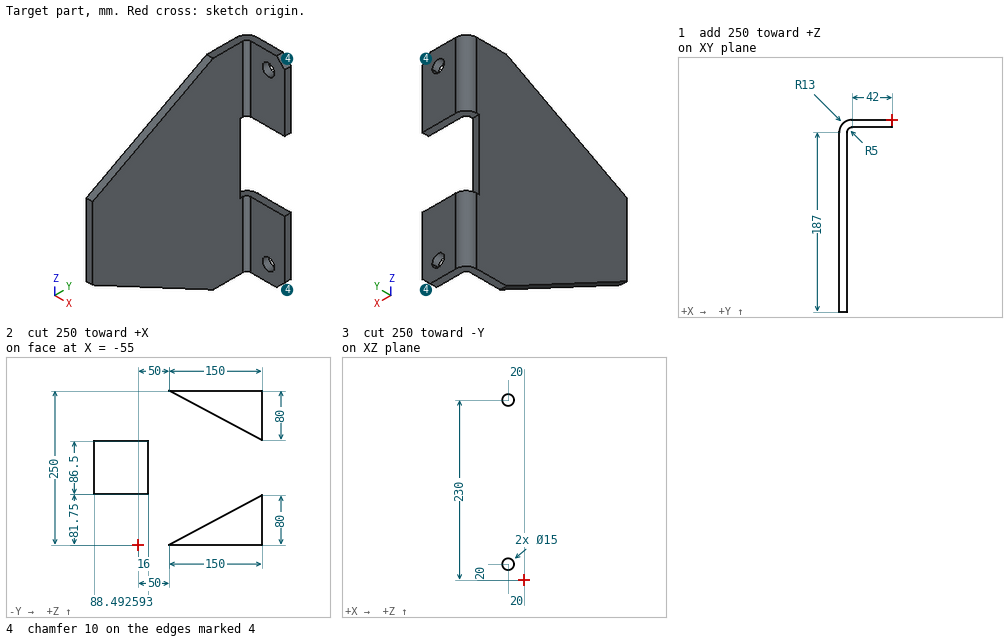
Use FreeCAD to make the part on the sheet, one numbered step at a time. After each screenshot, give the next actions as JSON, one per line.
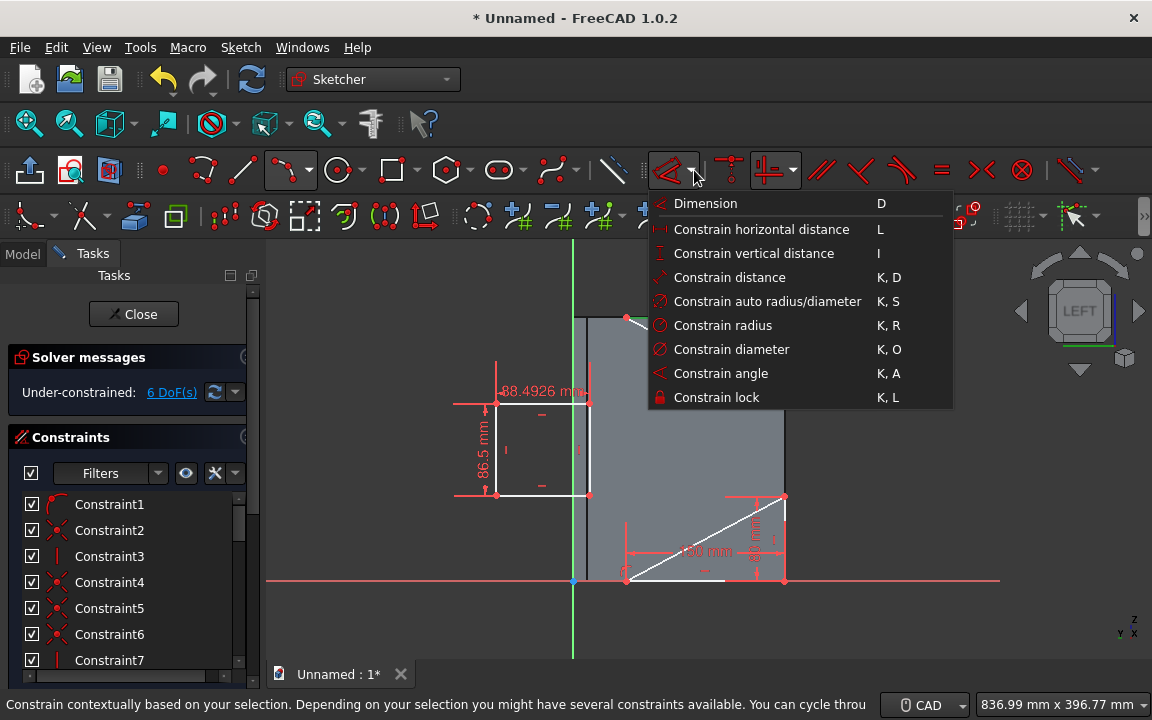
{"action": "left_click", "coordinate": [801, 229]}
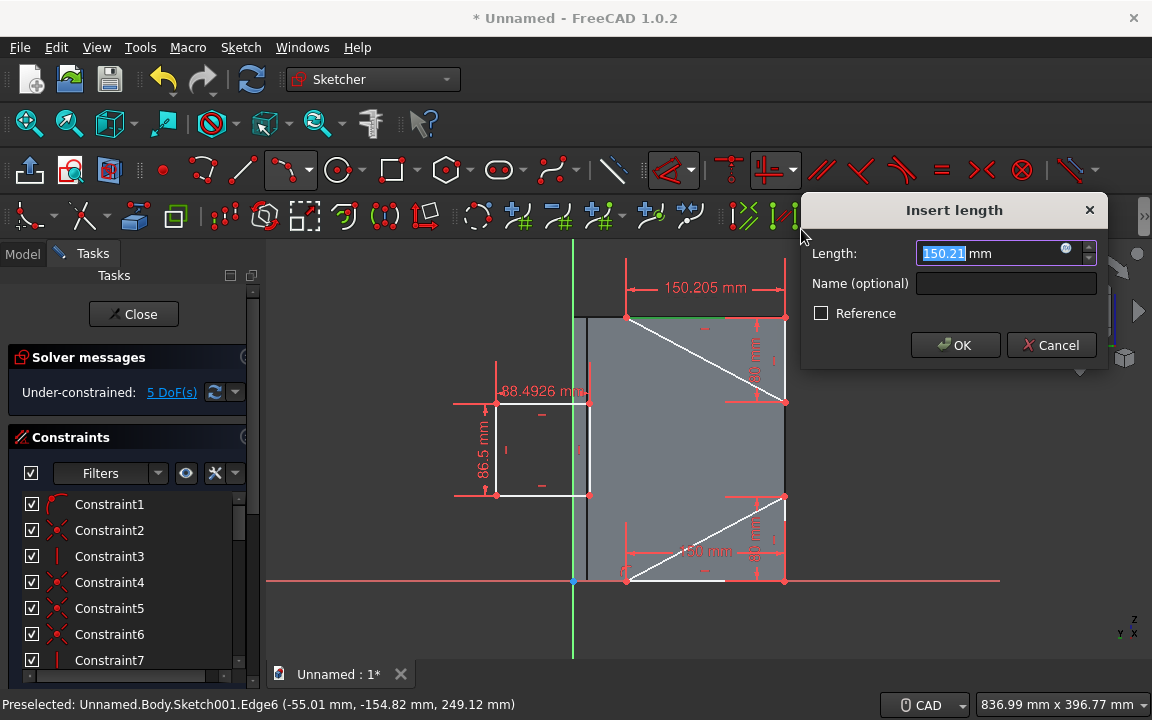
{"action": "type", "text": "150"}
{"action": "key", "text": "Return"}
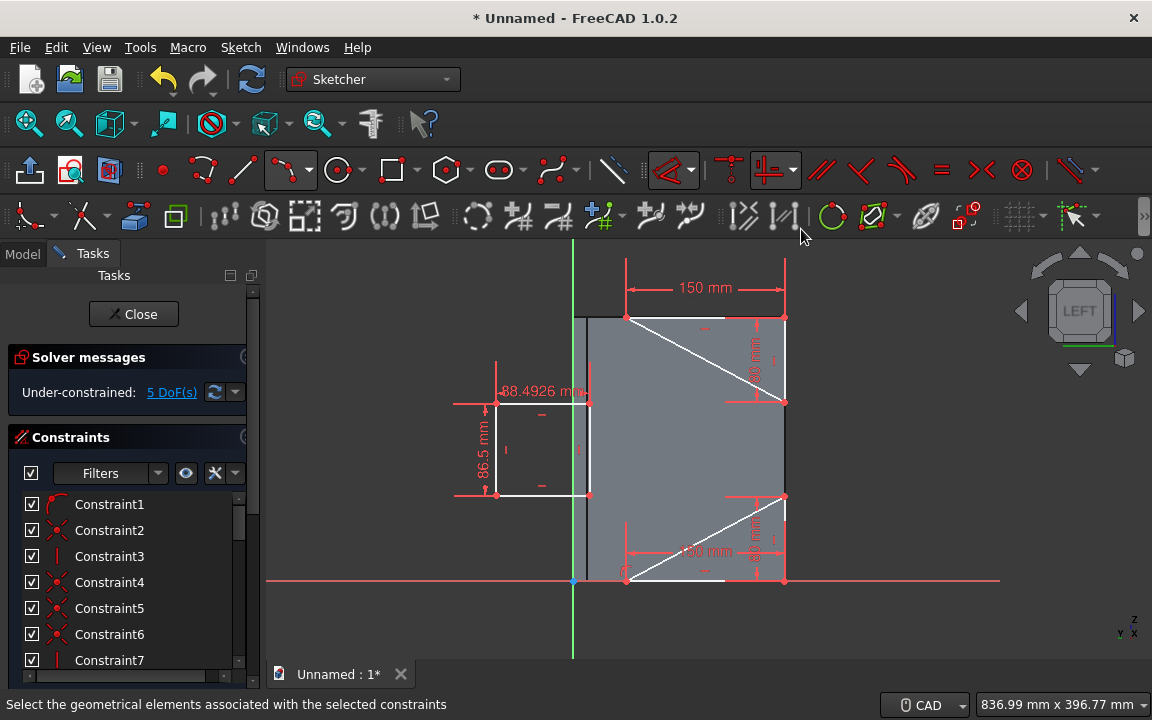
{"action": "left_click", "coordinate": [626, 581]}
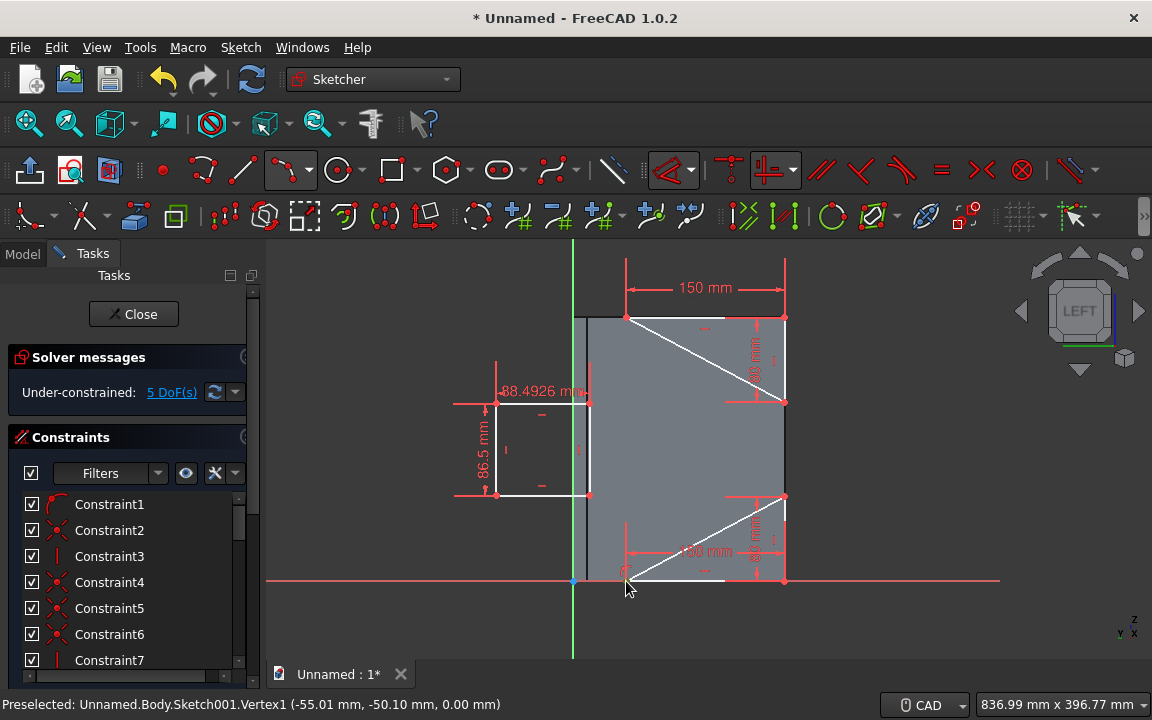
{"action": "key", "text": "l"}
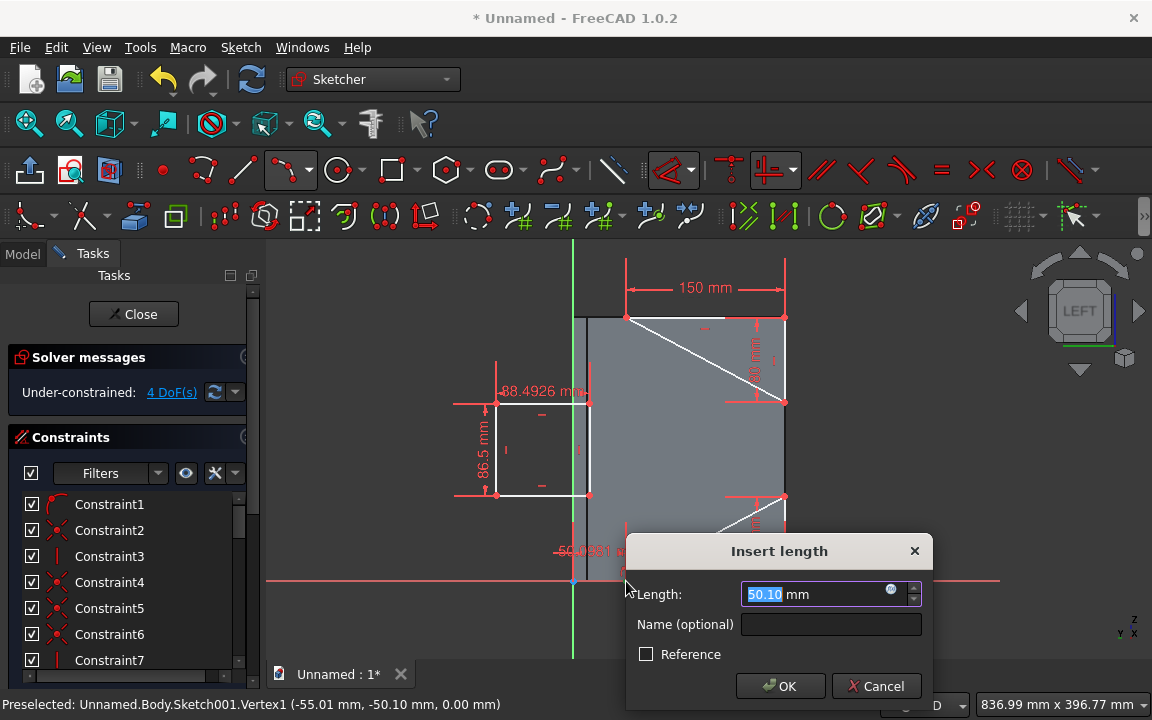
{"action": "type", "text": "50"}
{"action": "key", "text": "Return"}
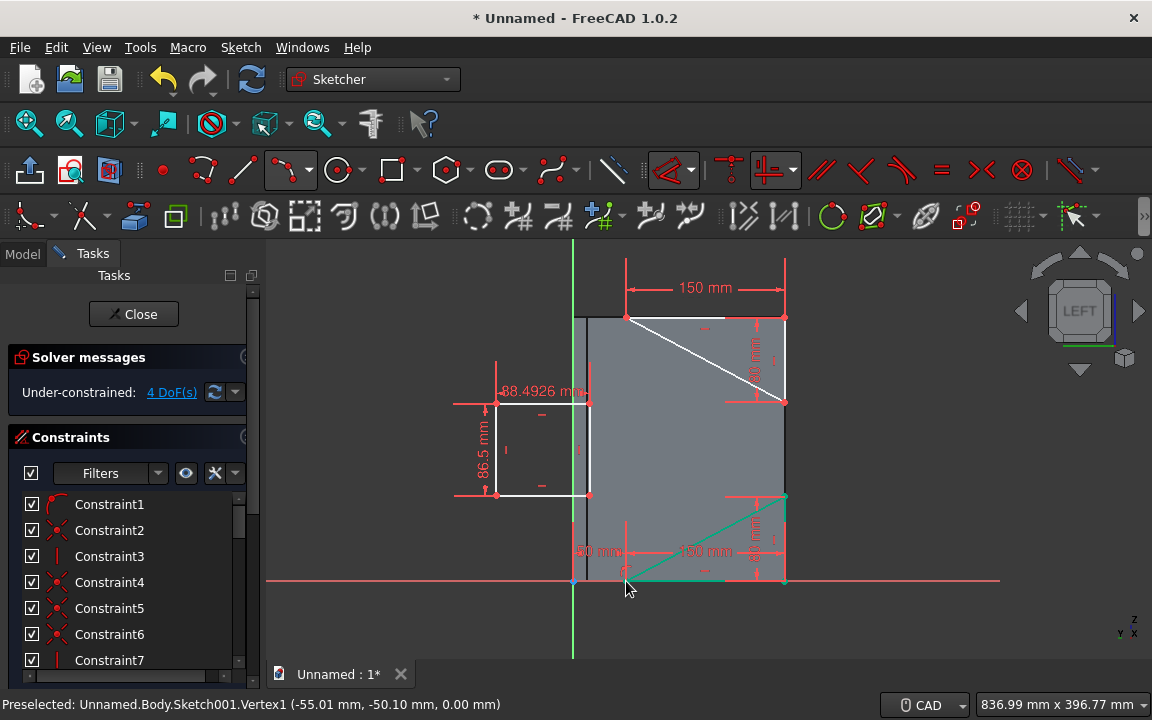
{"action": "left_click", "coordinate": [626, 318]}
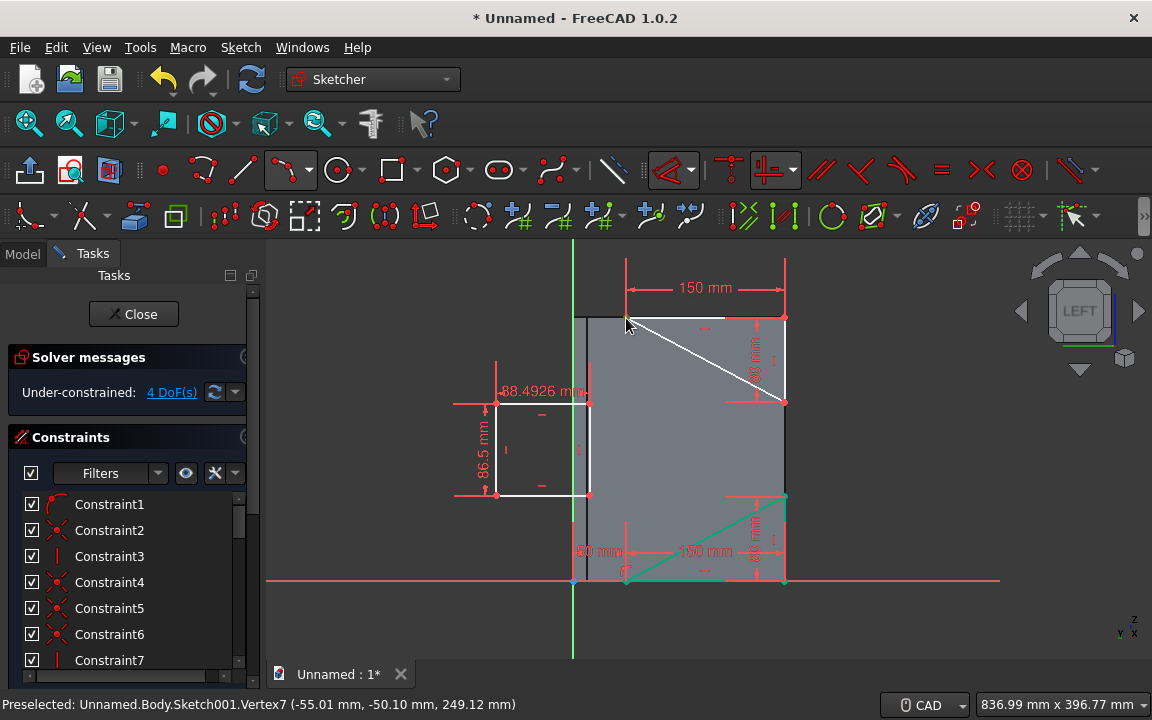
{"action": "key", "text": "l"}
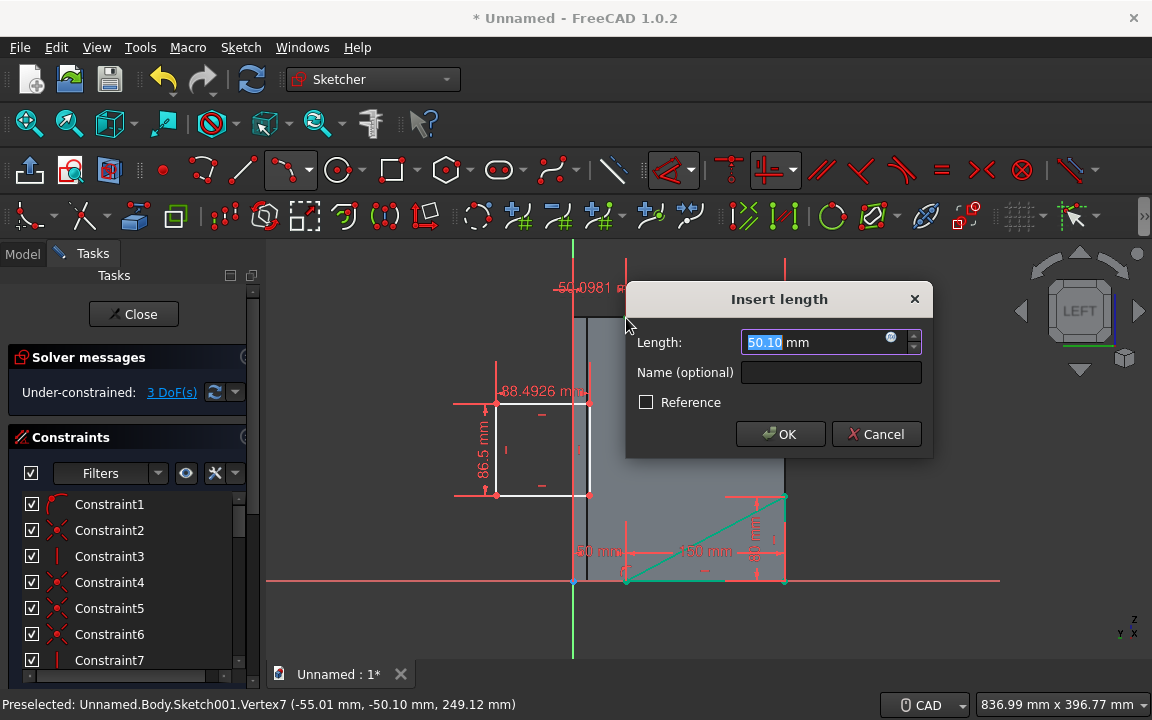
{"action": "type", "text": "50"}
{"action": "key", "text": "Return"}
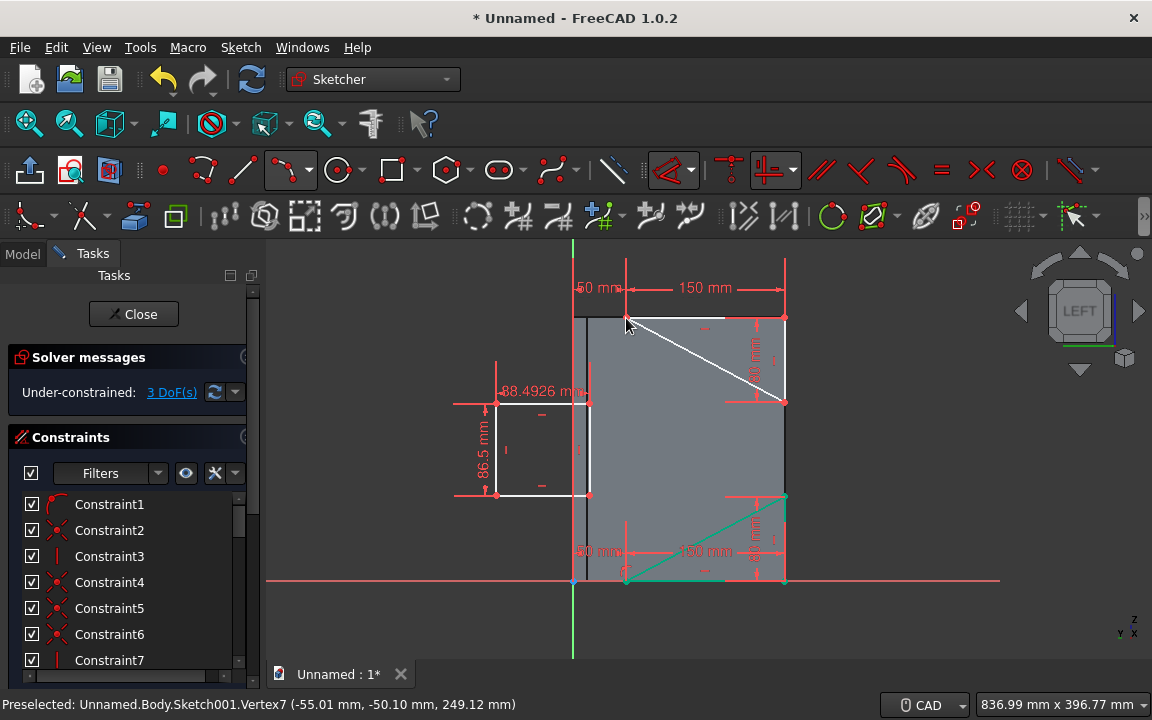
{"action": "scroll", "coordinate": [590, 496], "scroll_direction": "up", "scroll_amount": 5}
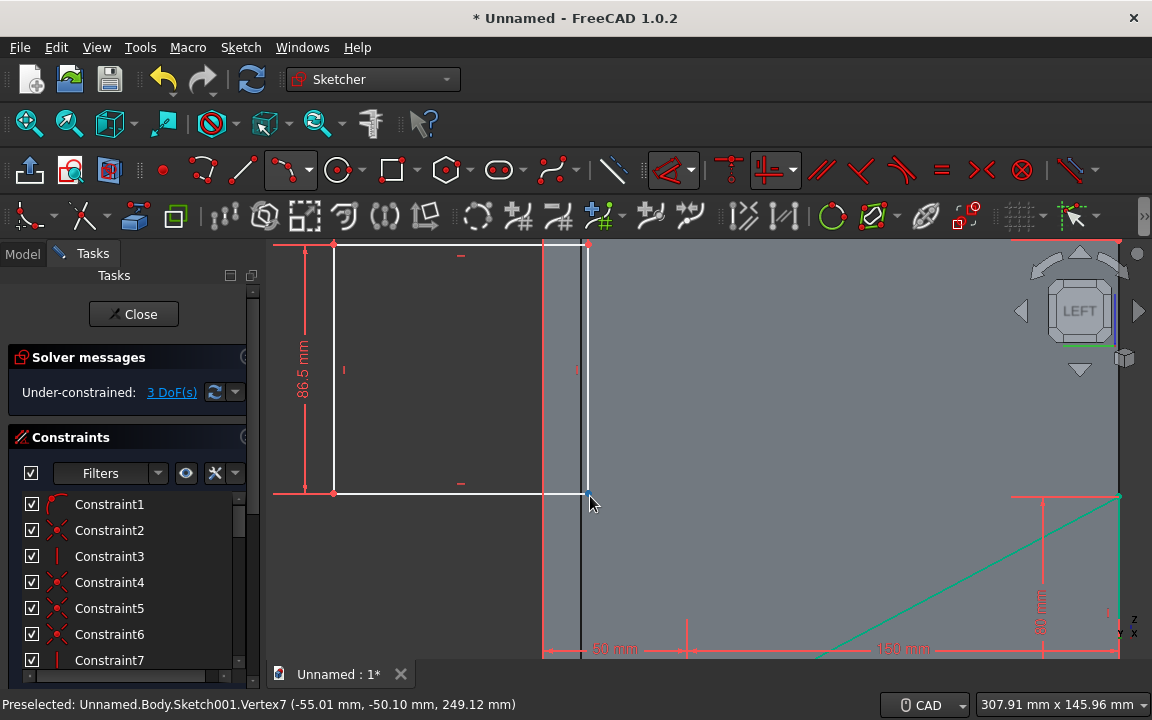
{"action": "left_click", "coordinate": [588, 494]}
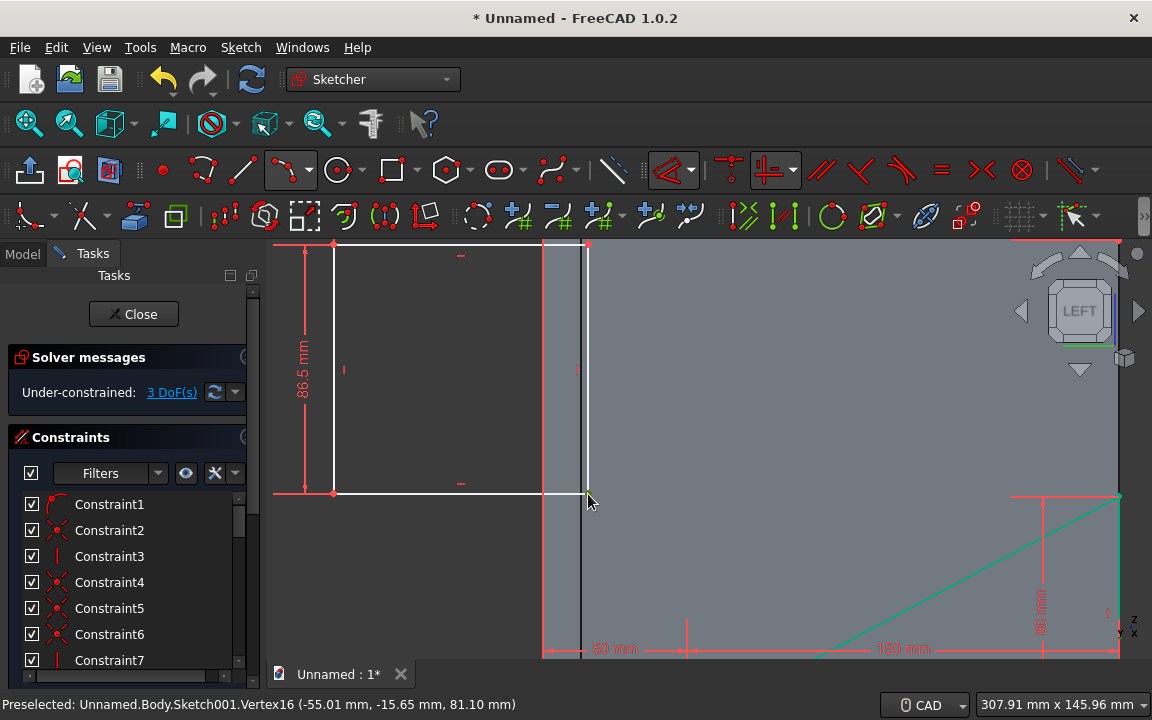
{"action": "key", "text": "l"}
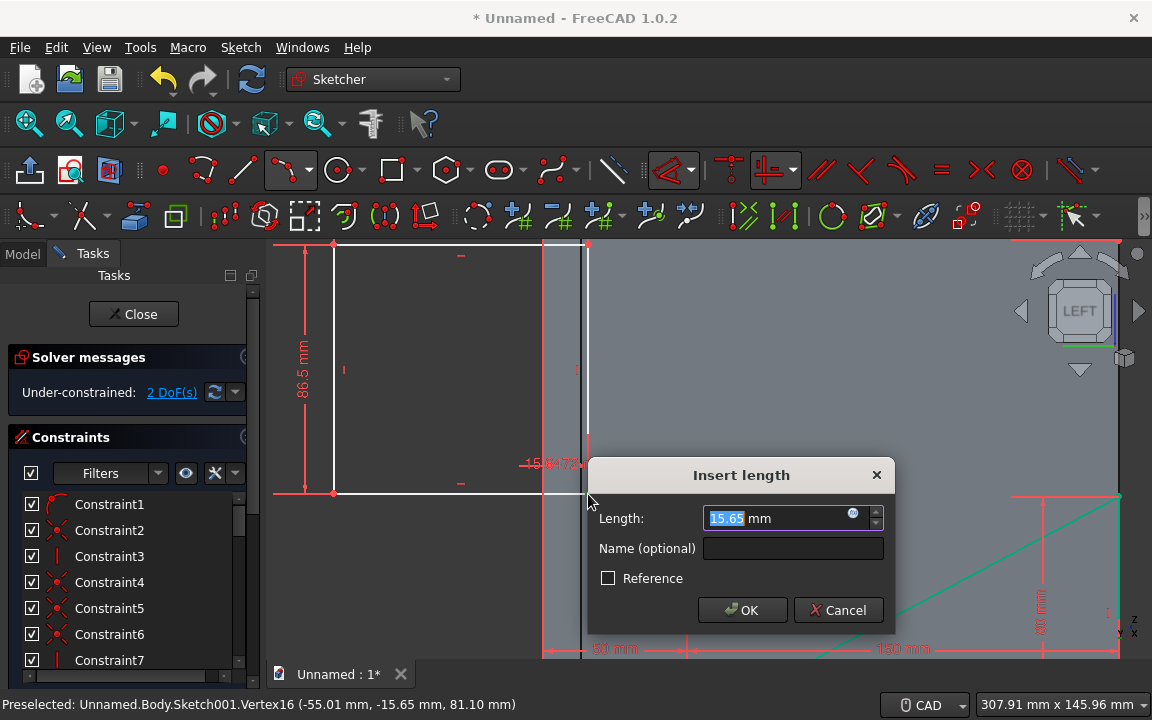
{"action": "type", "text": "16"}
{"action": "key", "text": "Return"}